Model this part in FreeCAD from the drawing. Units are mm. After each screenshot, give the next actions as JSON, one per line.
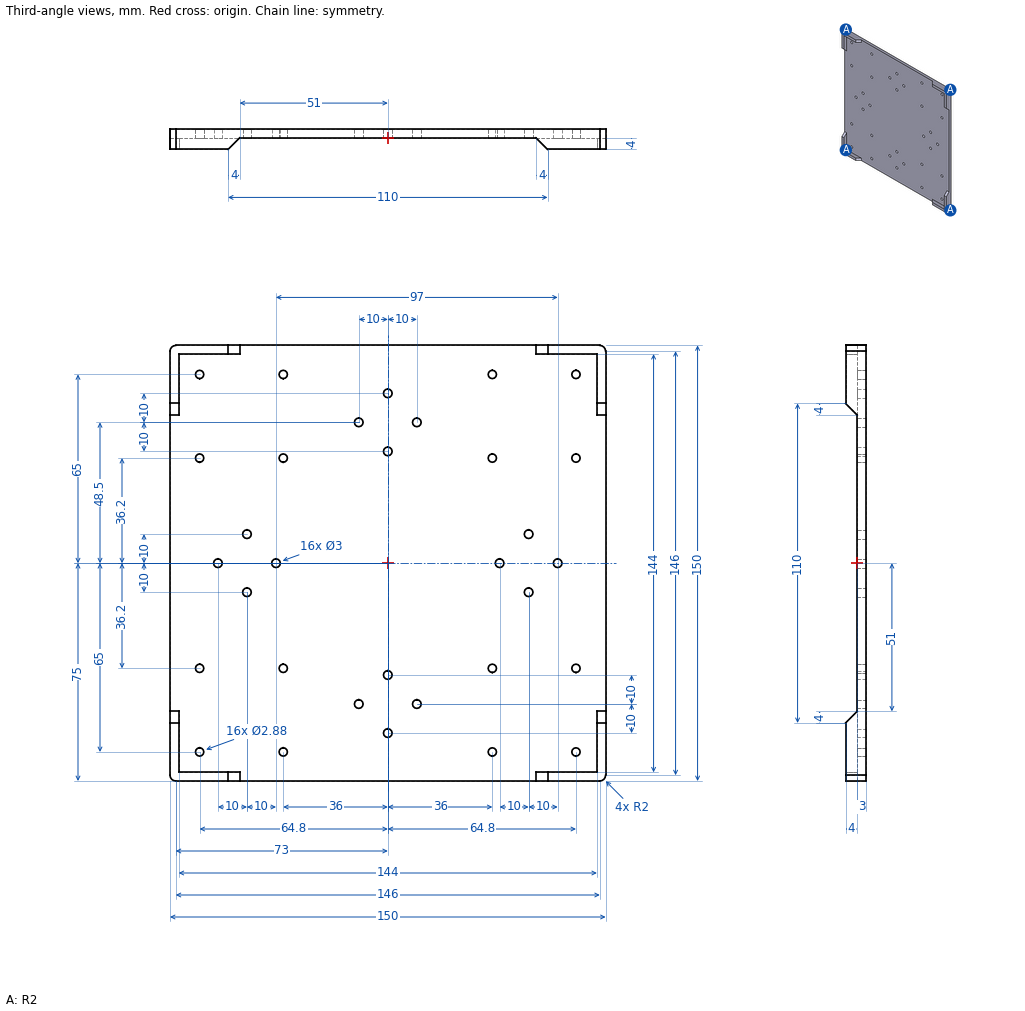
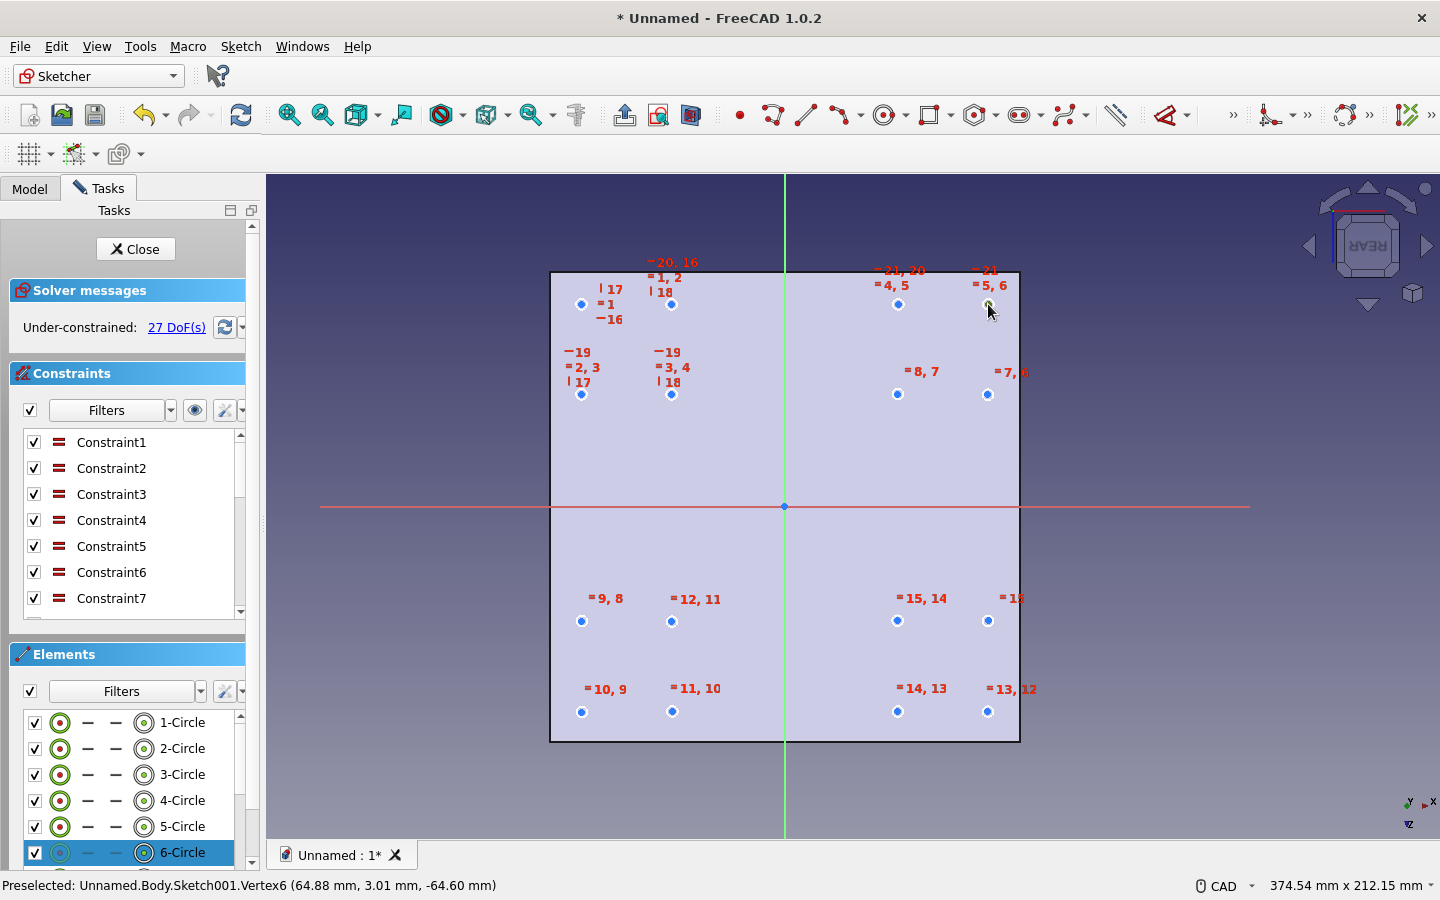
{"action": "left_click", "coordinate": [988, 395]}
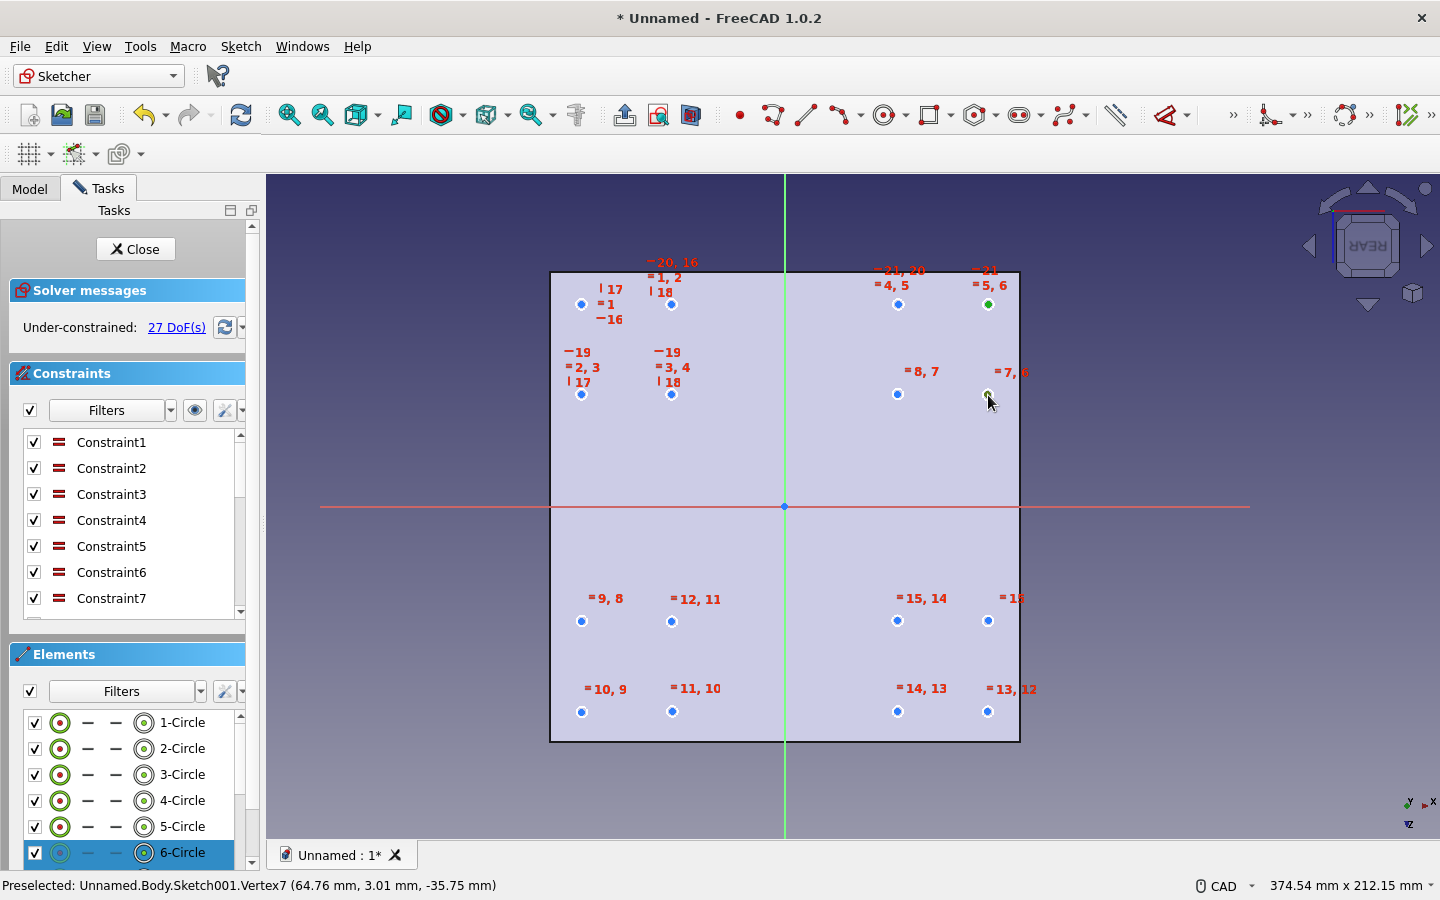
{"action": "key", "text": "v"}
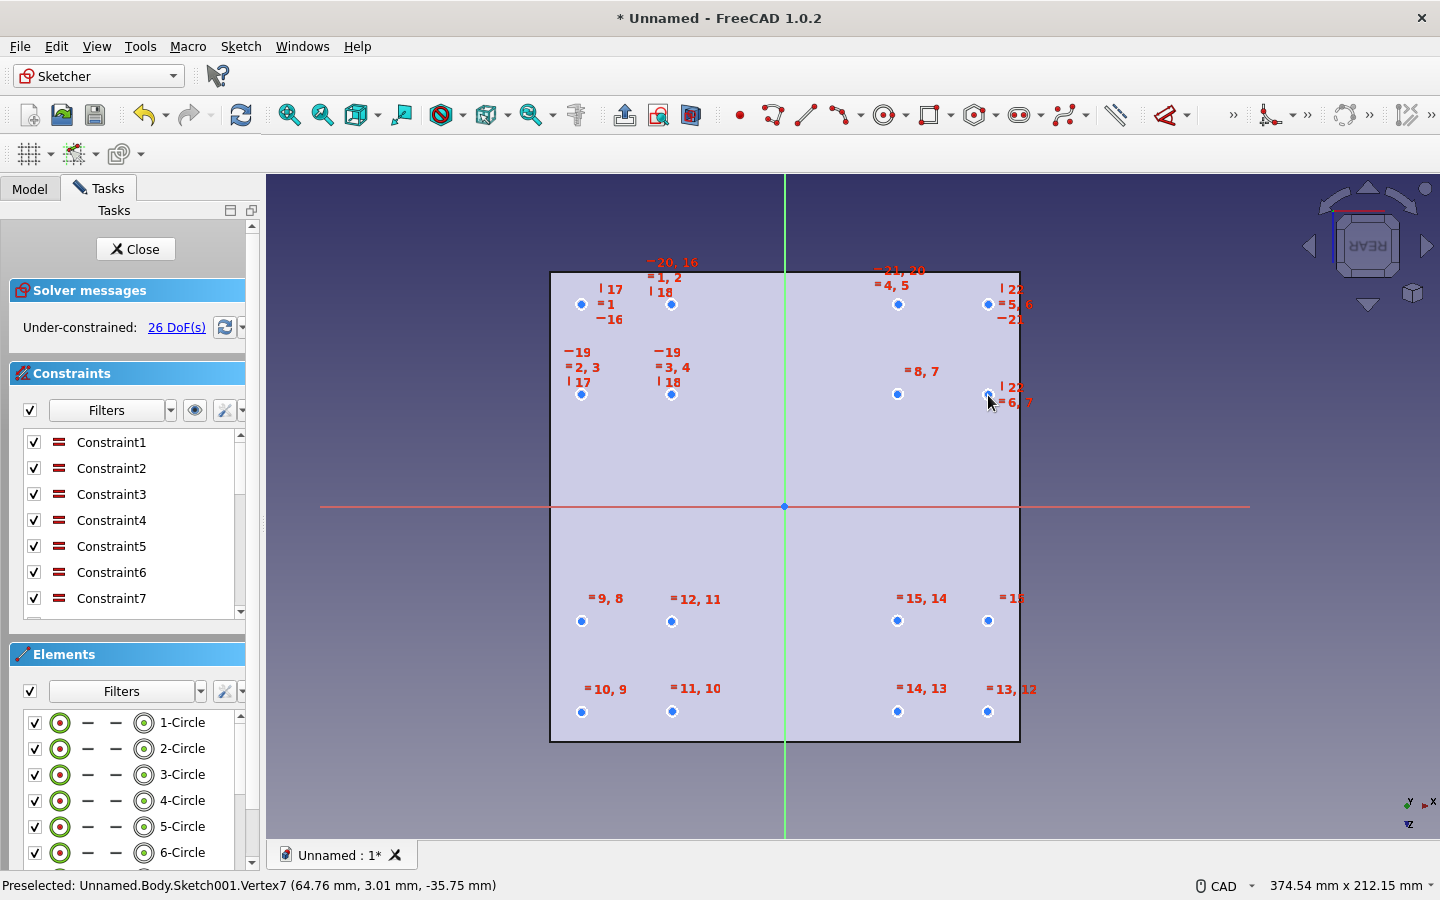
{"action": "left_click", "coordinate": [672, 394]}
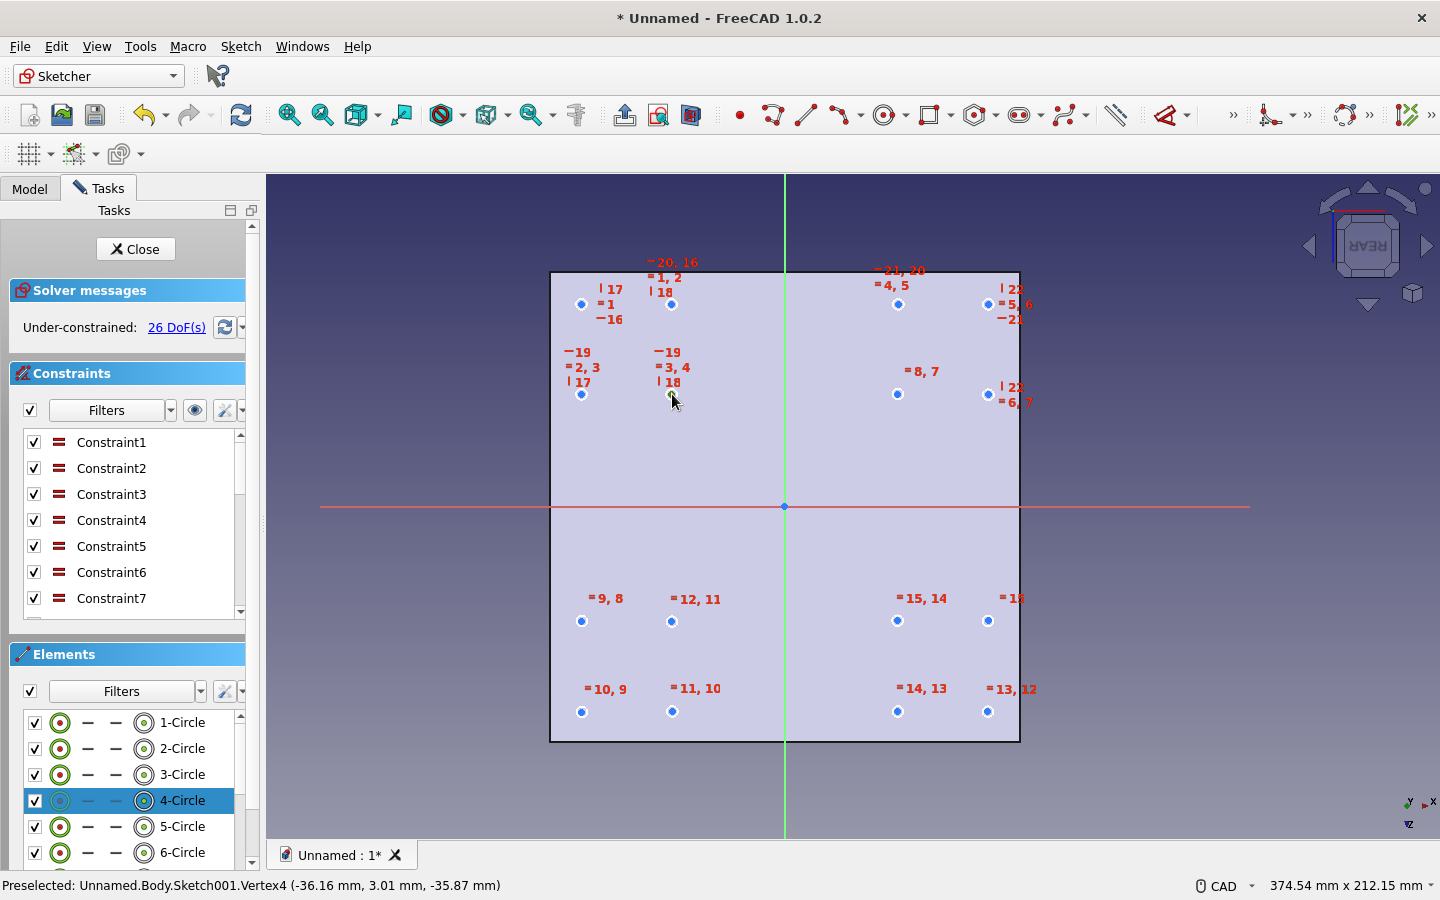
{"action": "left_click", "coordinate": [988, 395]}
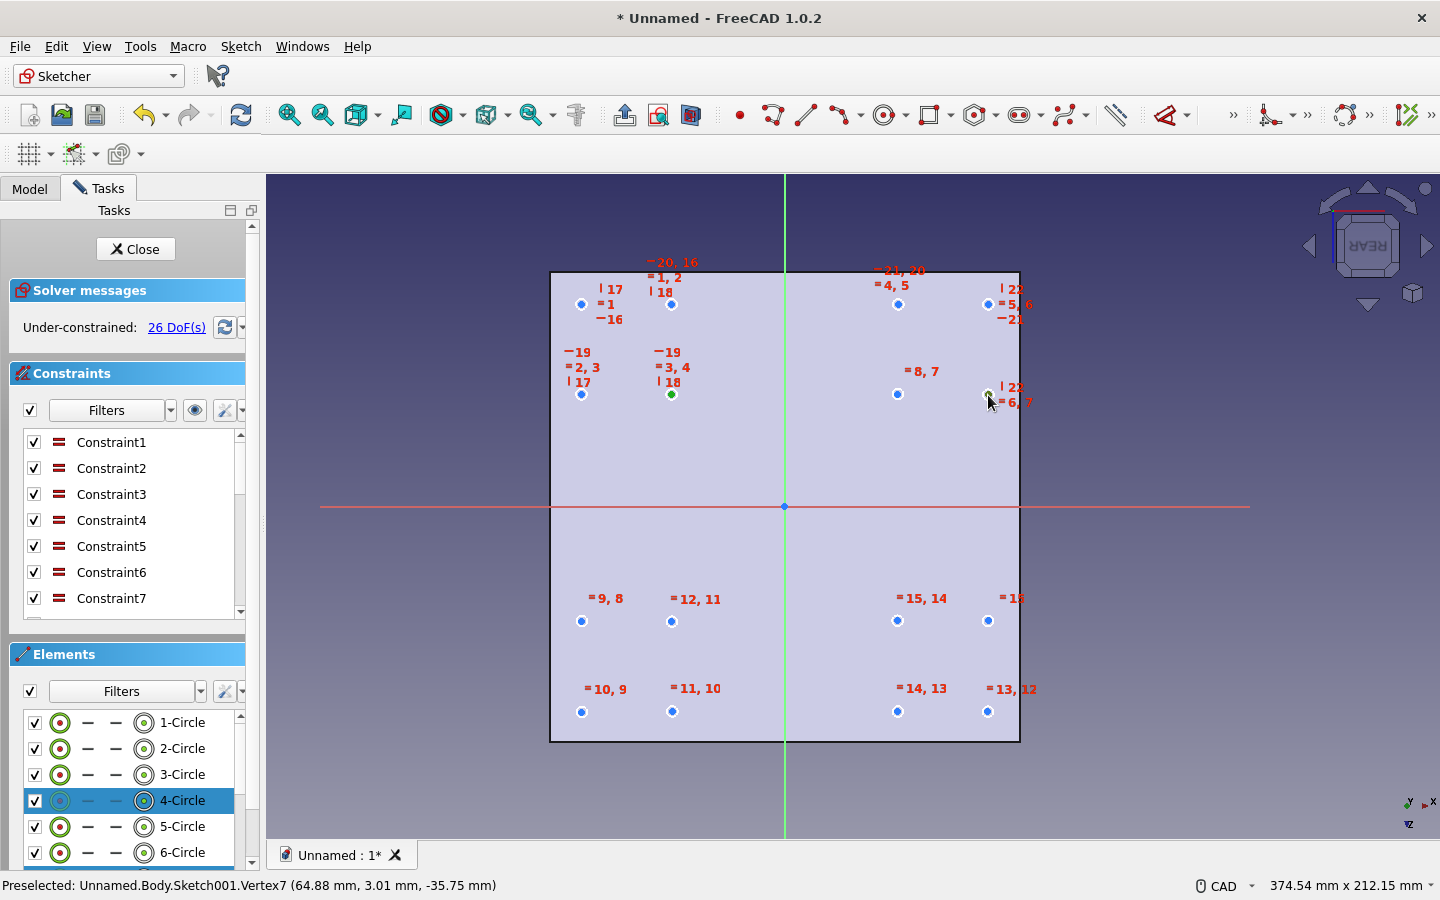
{"action": "key", "text": "h"}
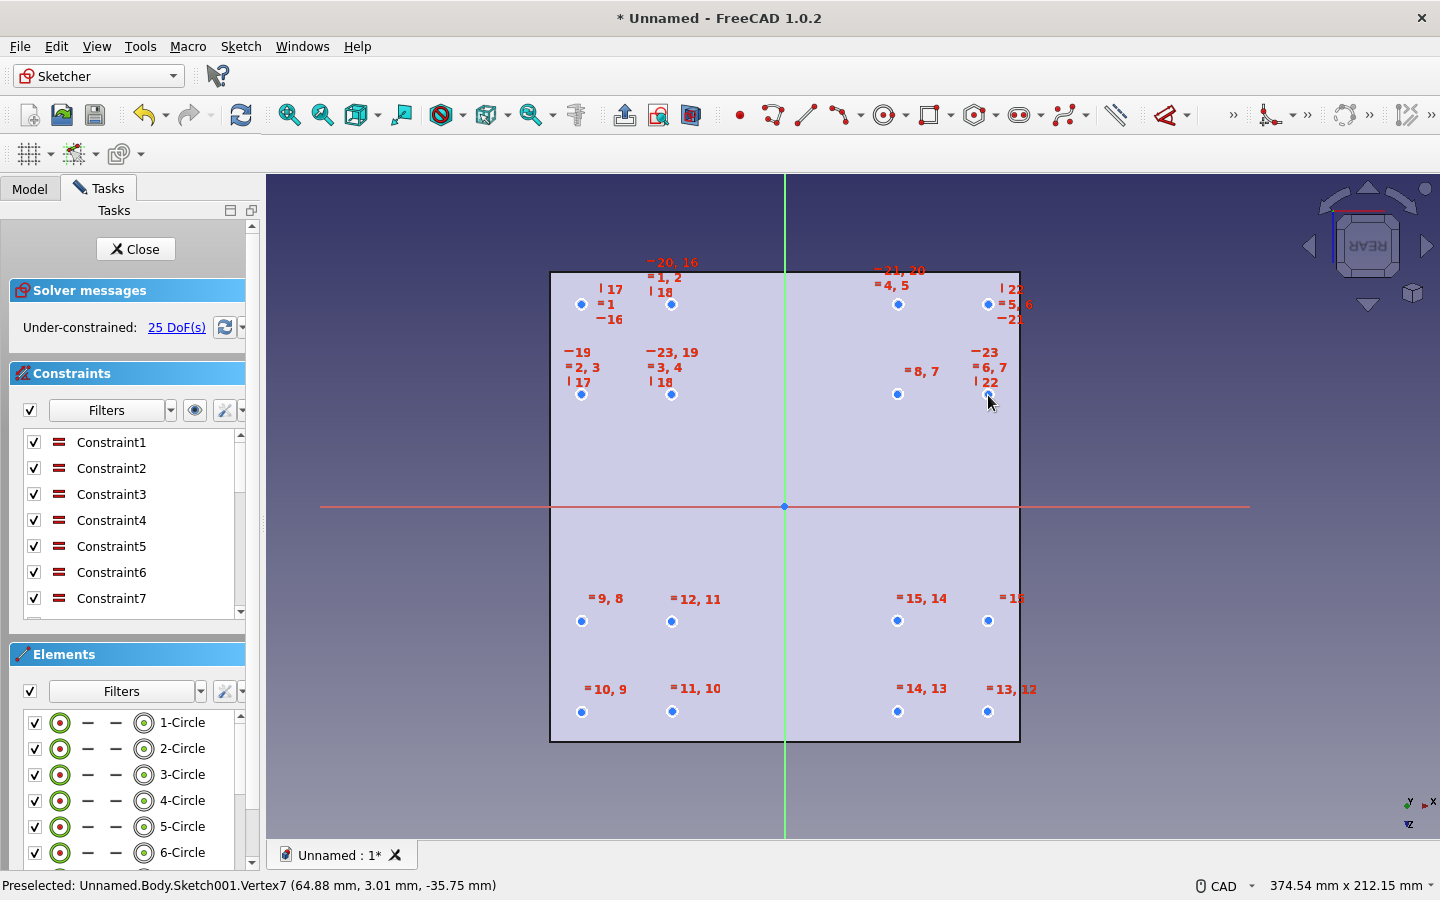
{"action": "left_click", "coordinate": [898, 304]}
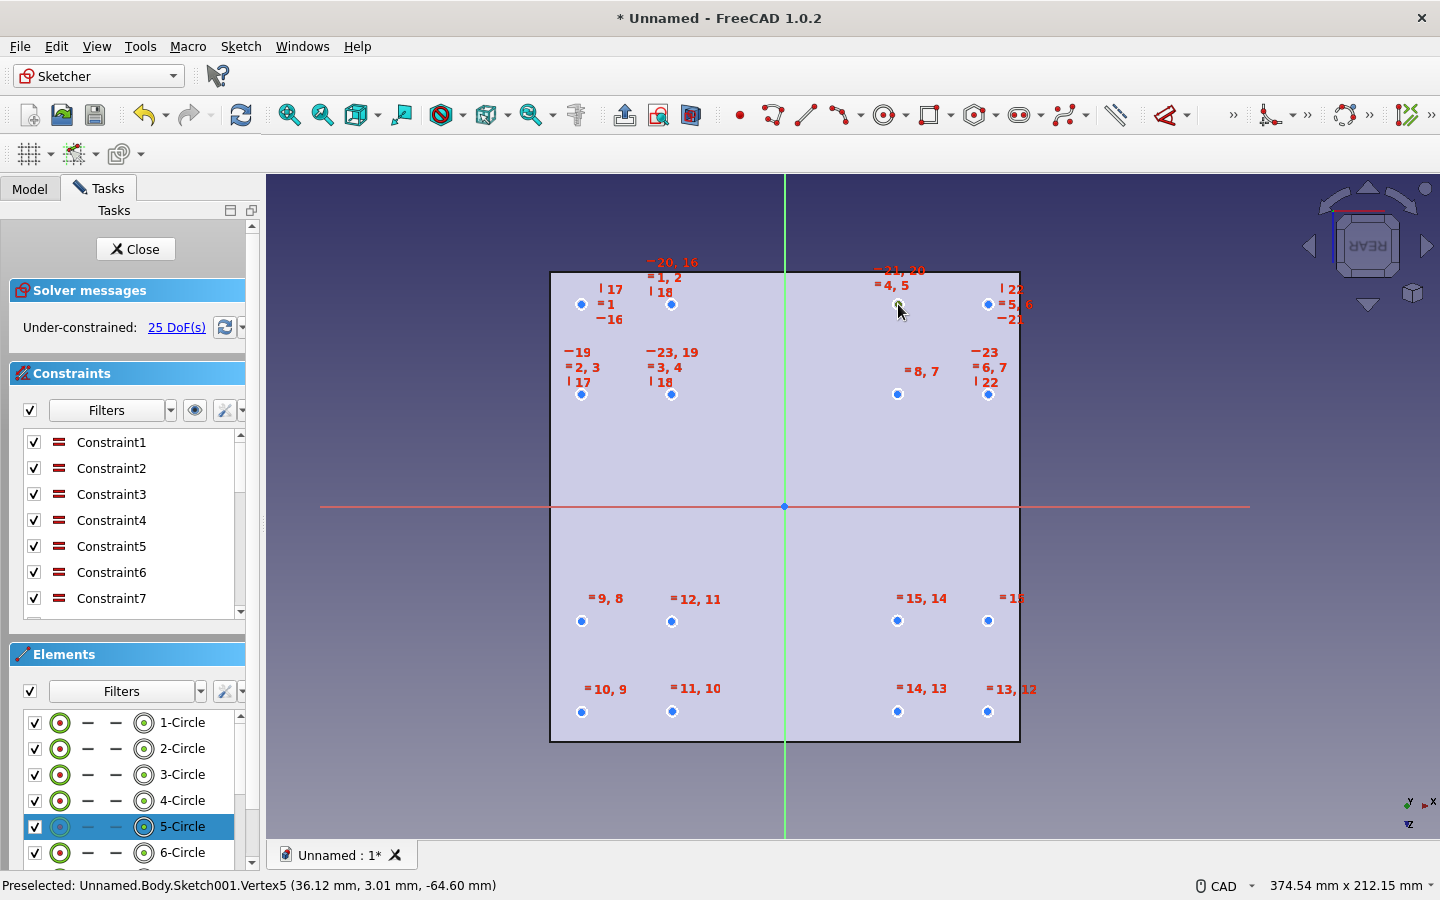
{"action": "left_click", "coordinate": [898, 394]}